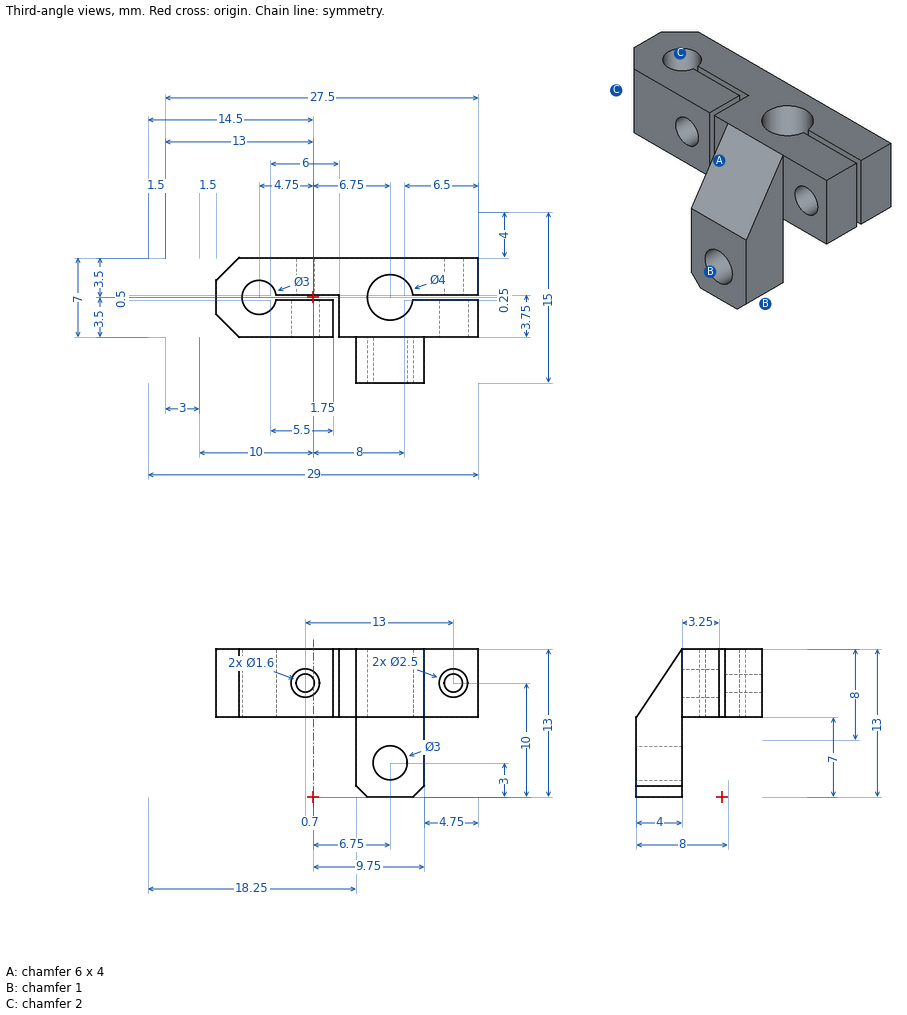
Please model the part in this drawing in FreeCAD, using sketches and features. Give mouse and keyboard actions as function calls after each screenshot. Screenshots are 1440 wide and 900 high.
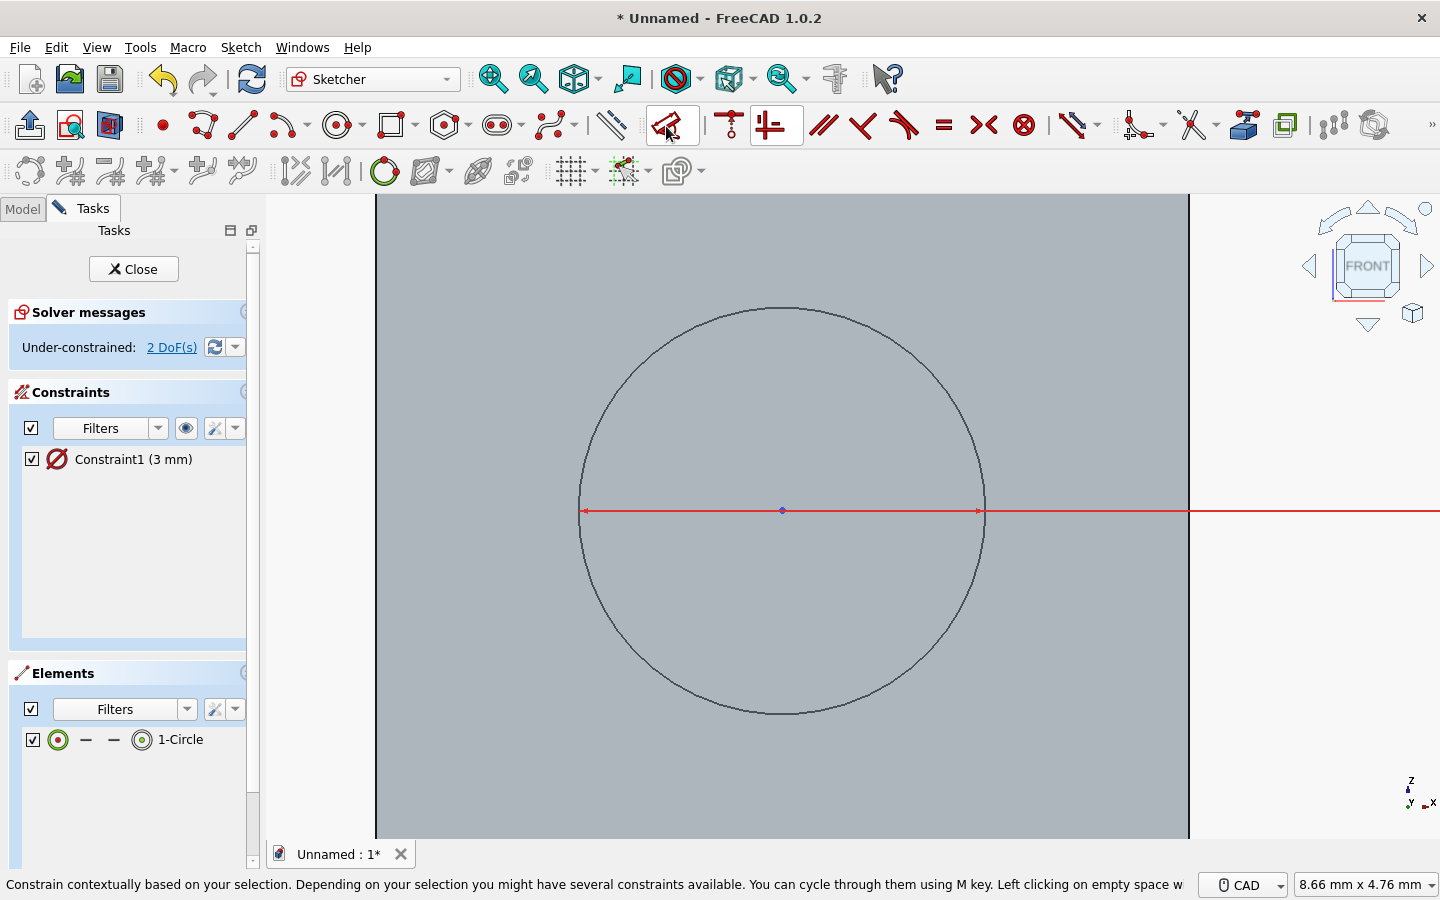
click(782, 511)
click(816, 661)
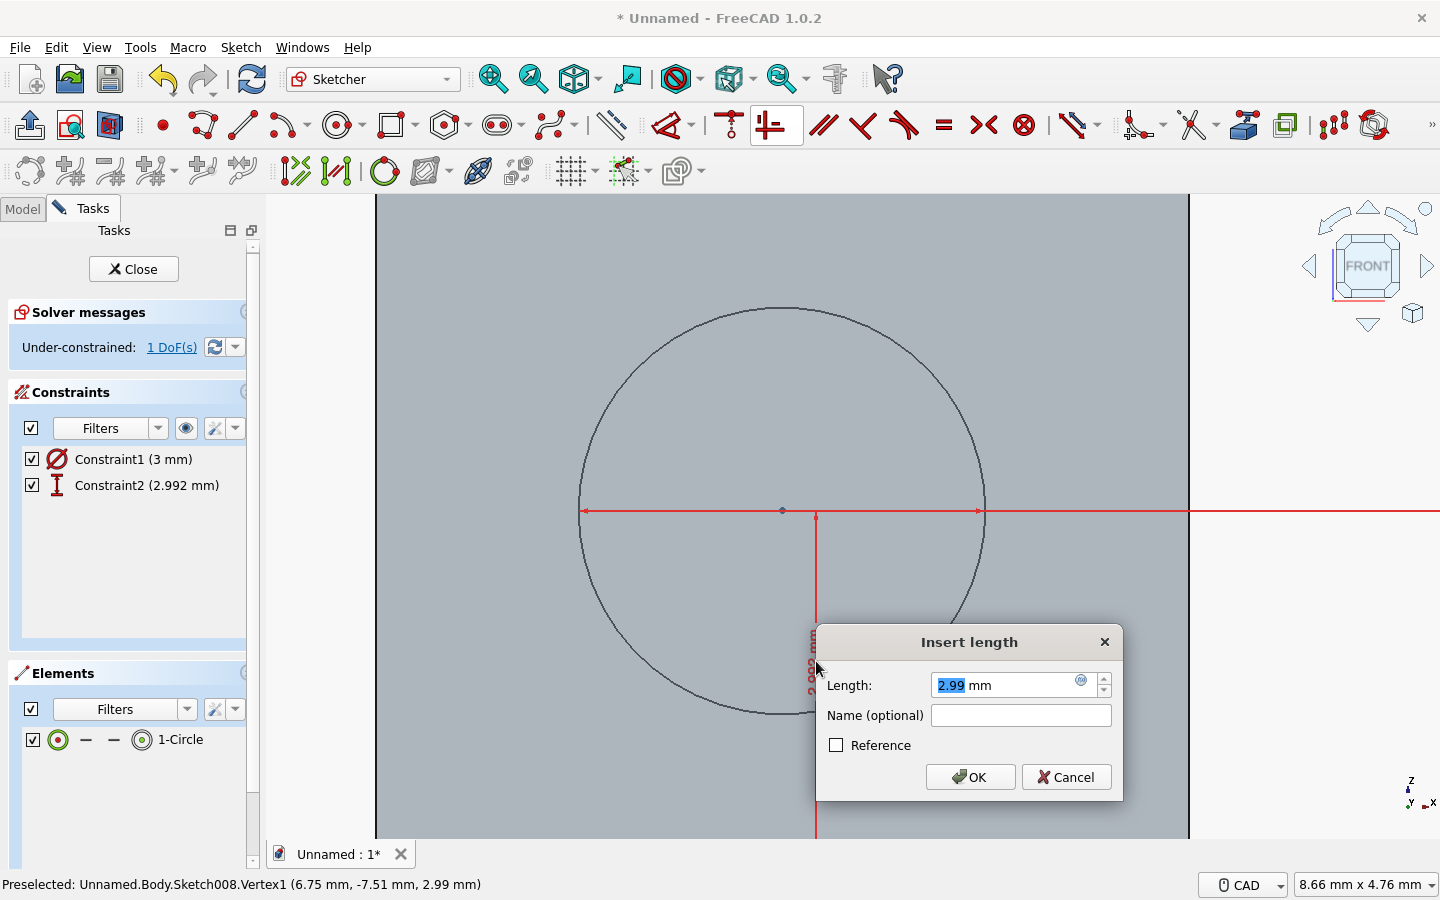
text(3)
key(Return)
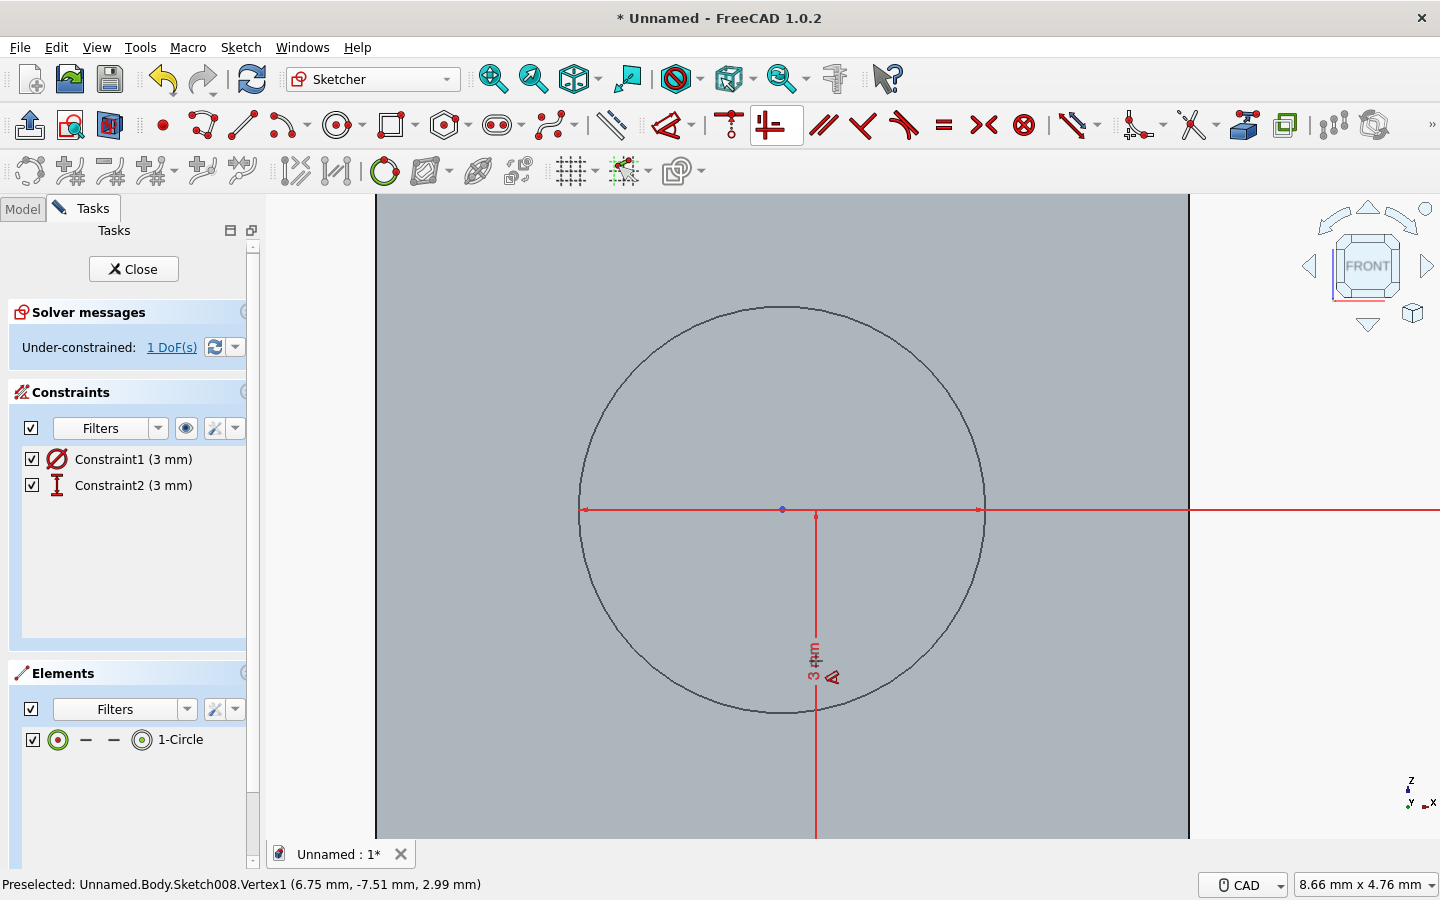
click(782, 510)
click(538, 476)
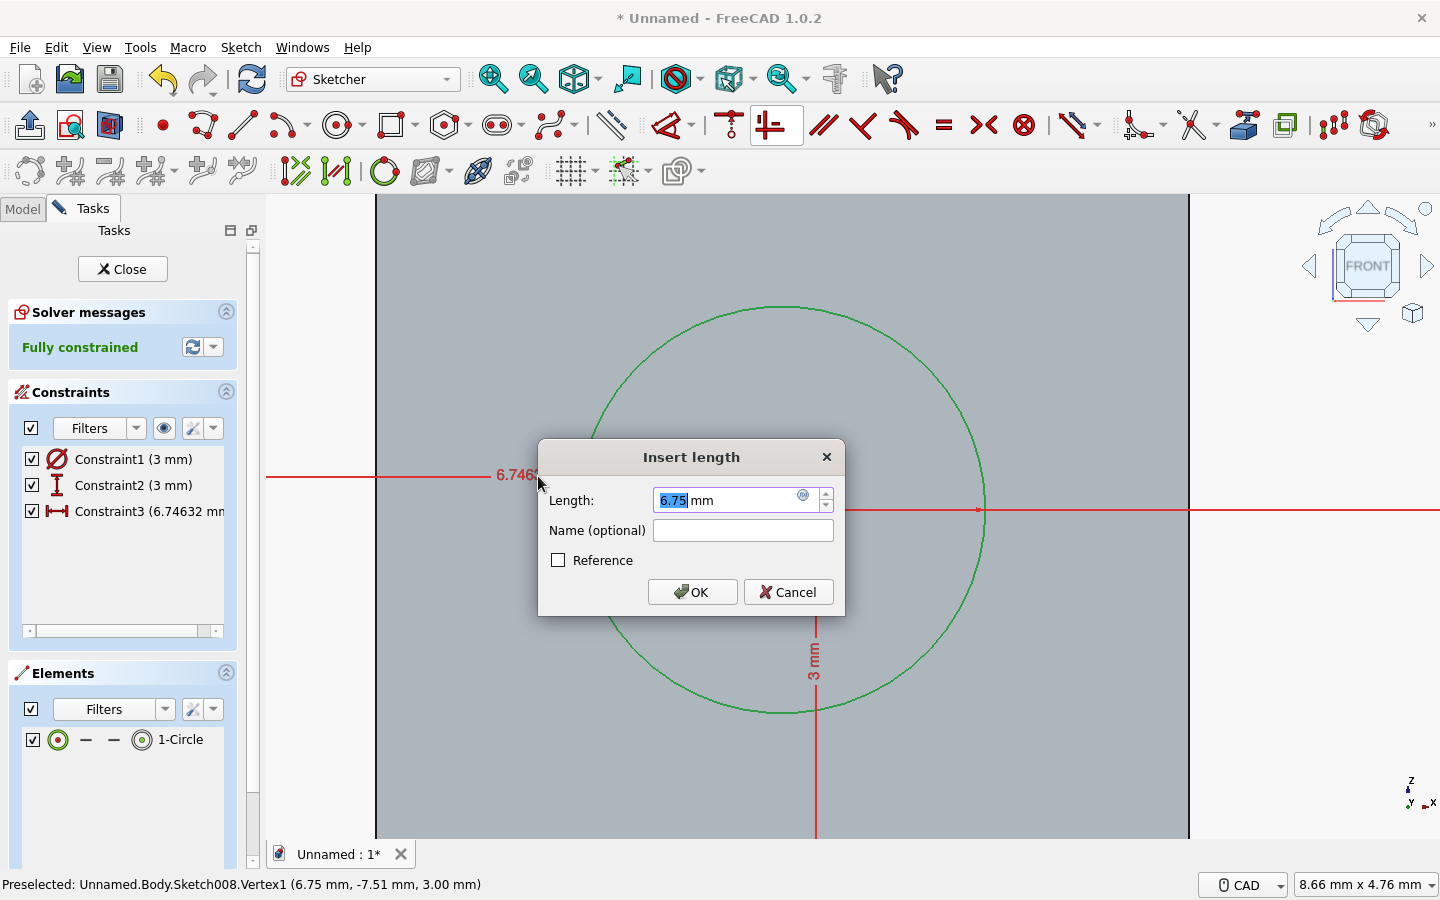
text(6.75)
key(Return)
key(Escape)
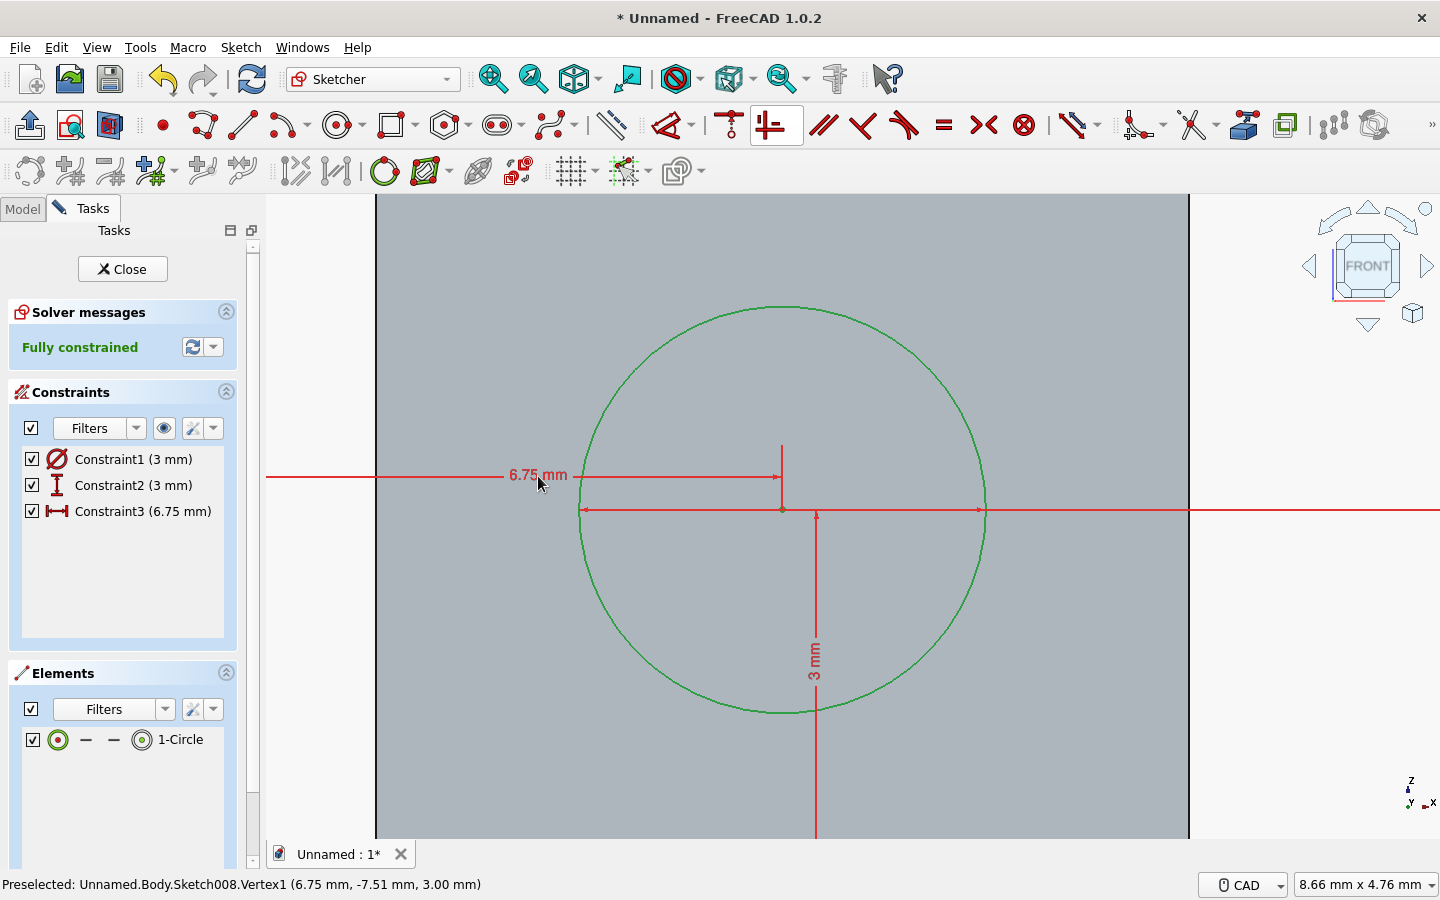
click(123, 269)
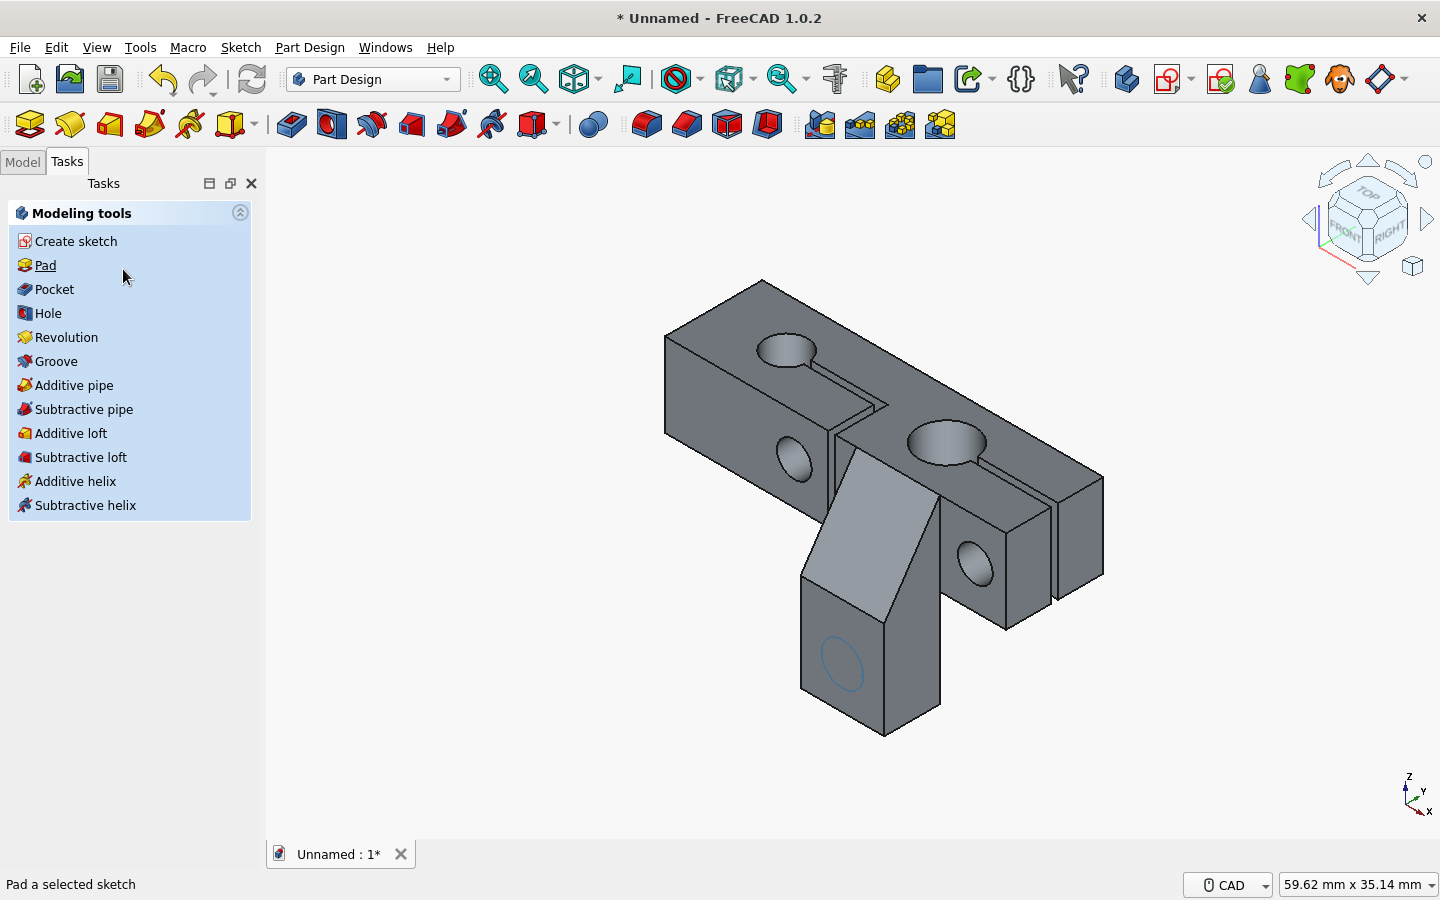
click(292, 124)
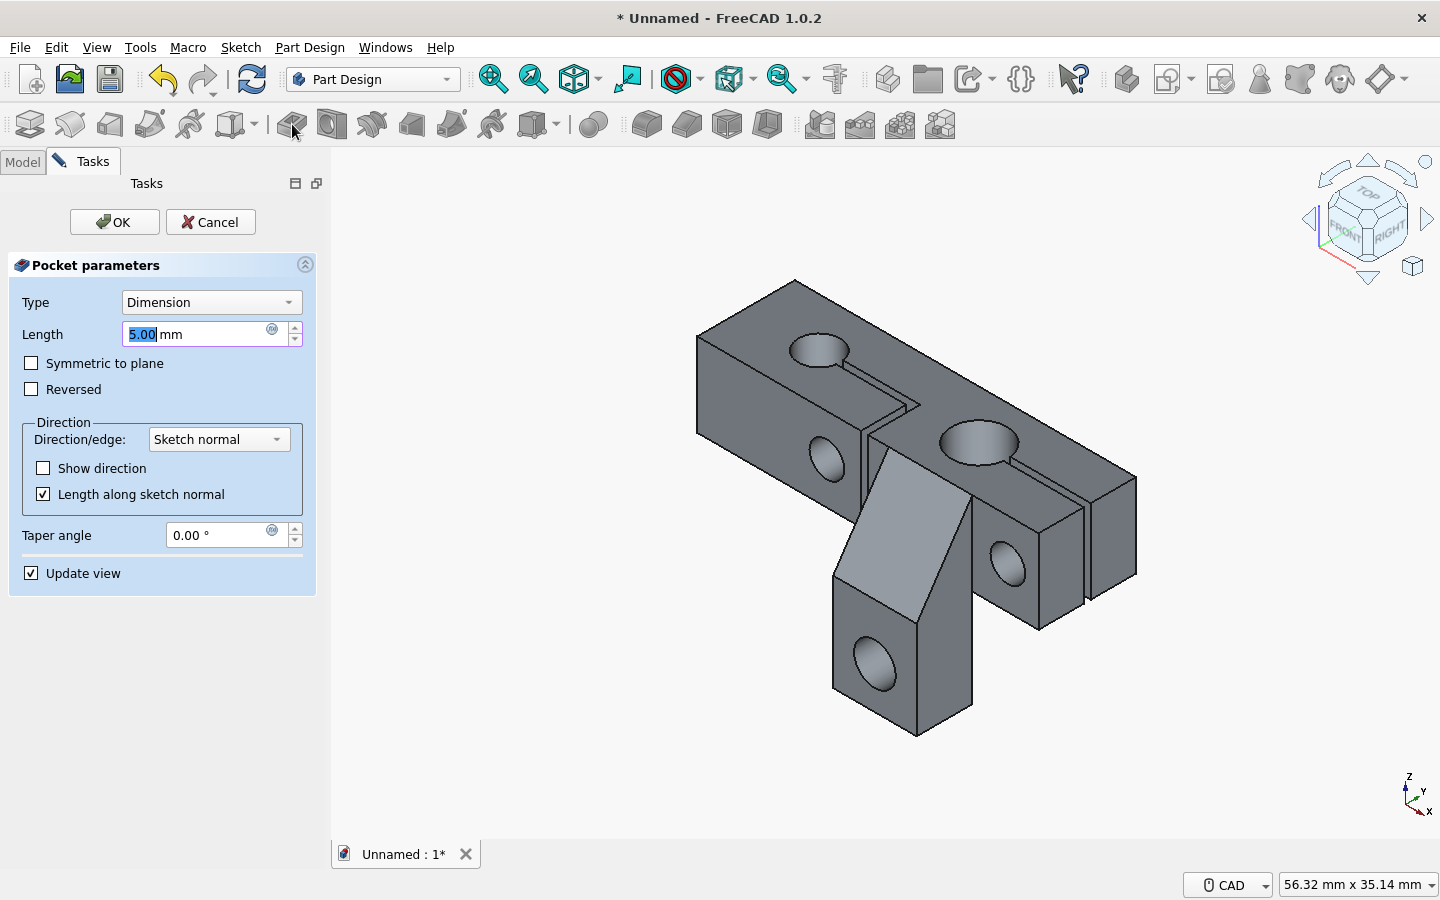
text(8)
key(Tab)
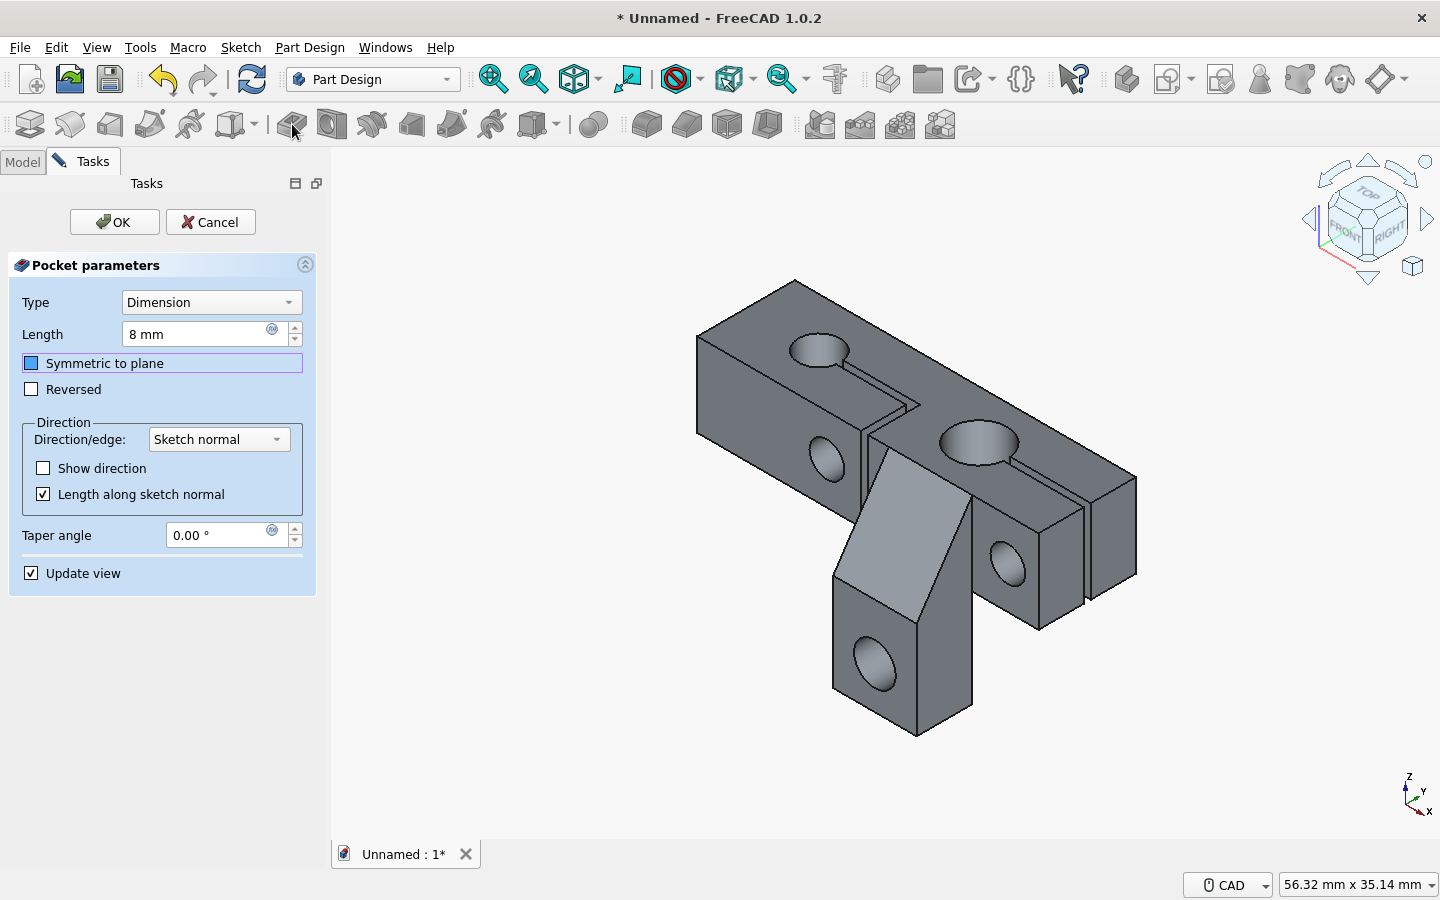
click(115, 222)